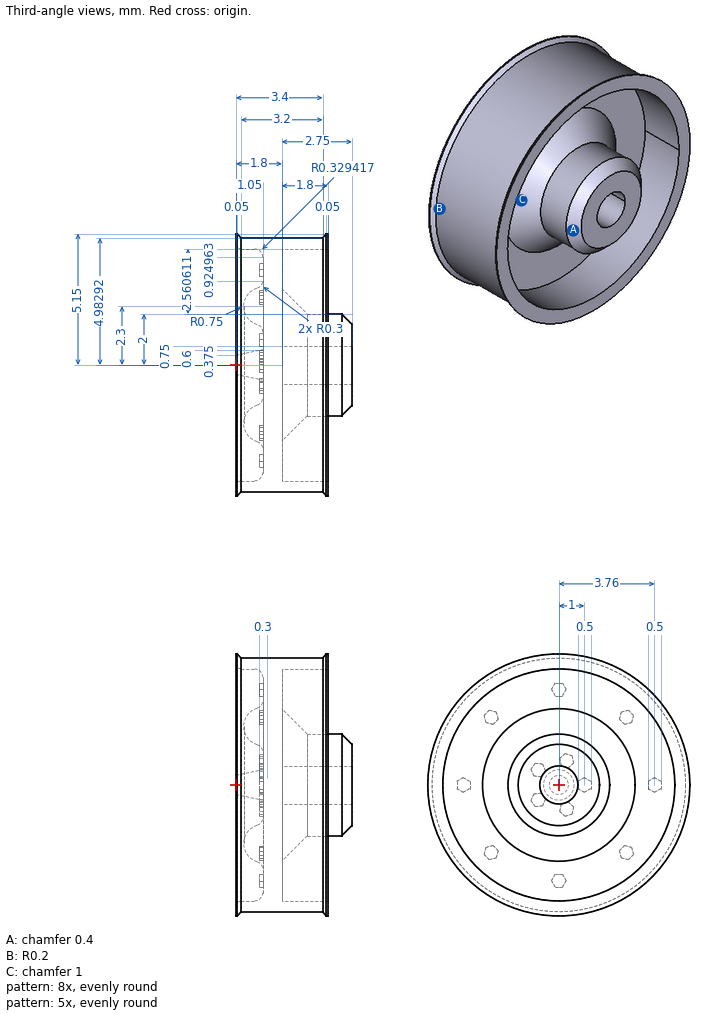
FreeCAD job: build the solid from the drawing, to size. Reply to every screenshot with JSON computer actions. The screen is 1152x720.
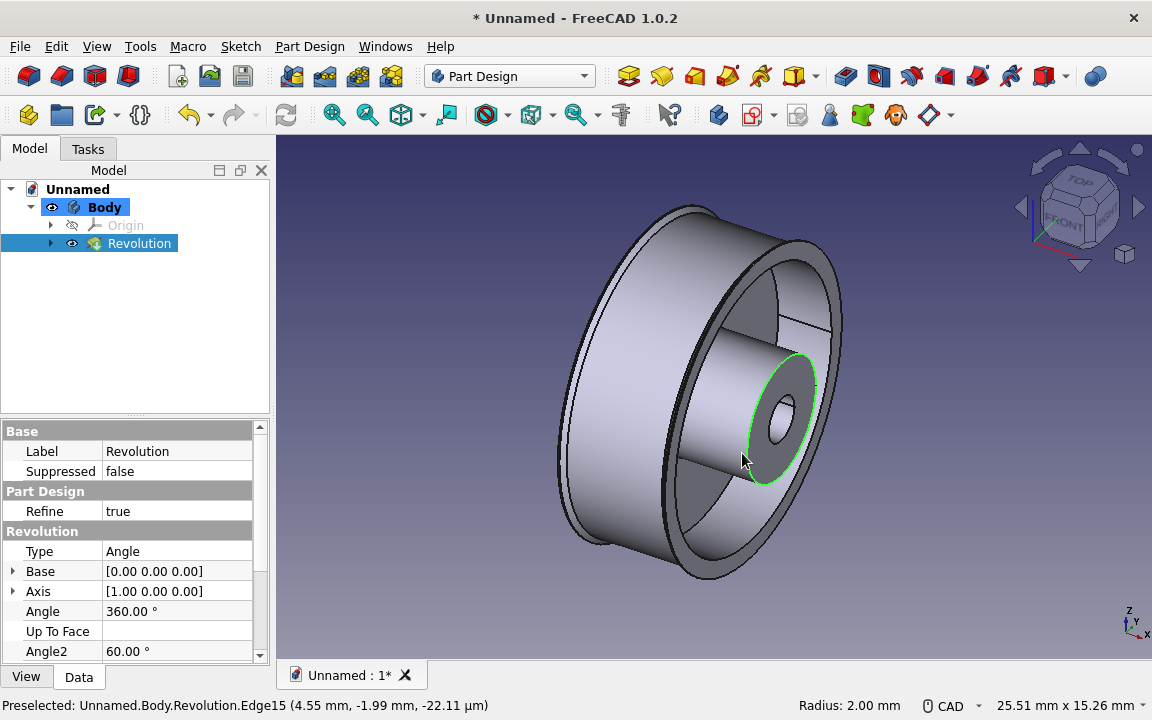
{"action": "left_click", "coordinate": [62, 76]}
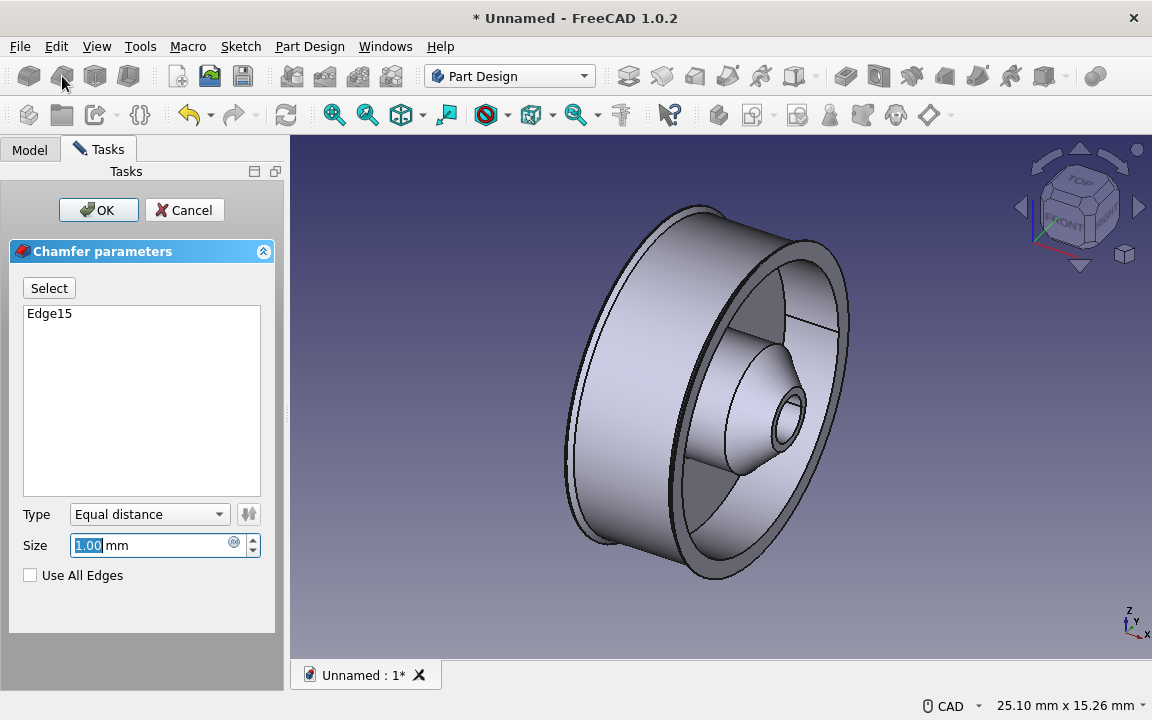
{"action": "type", "text": "0.4"}
{"action": "key", "text": "Tab"}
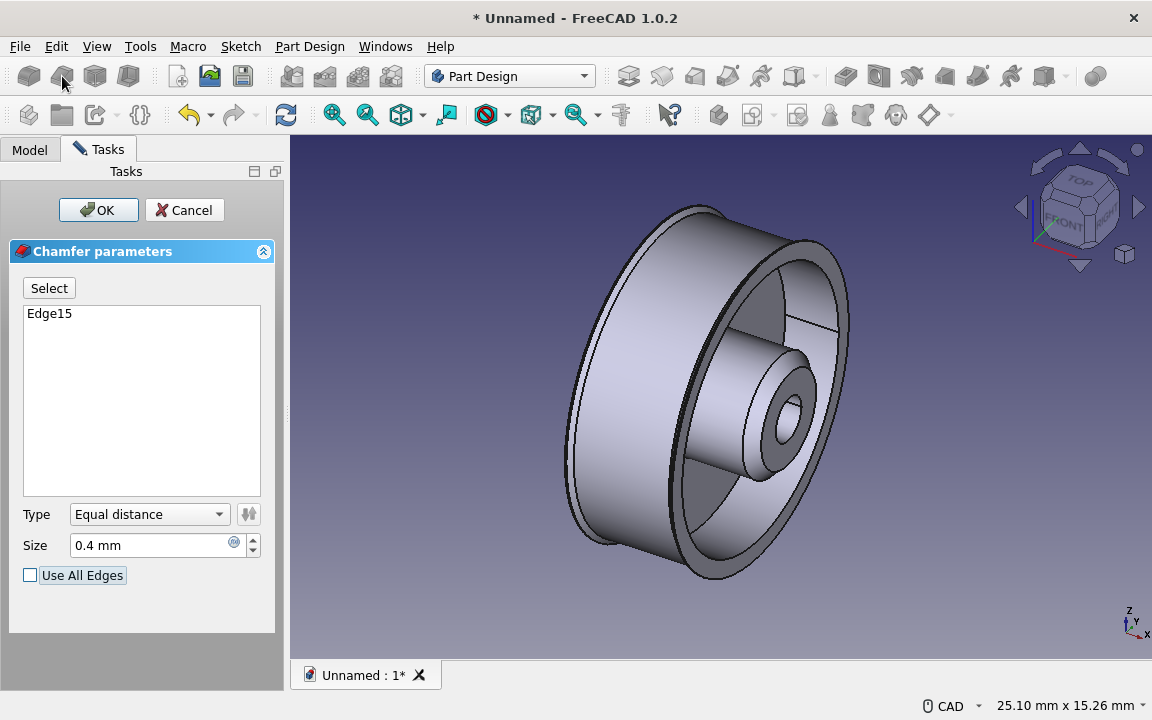
{"action": "left_click", "coordinate": [99, 210]}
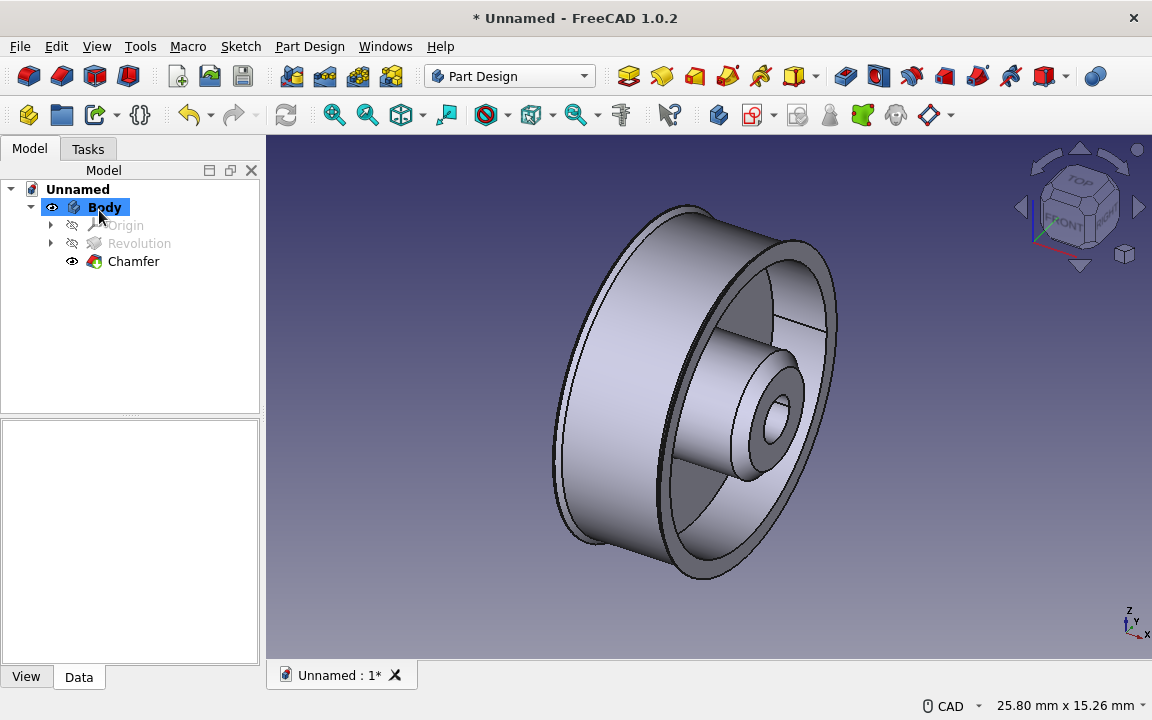
{"action": "key", "text": "0"}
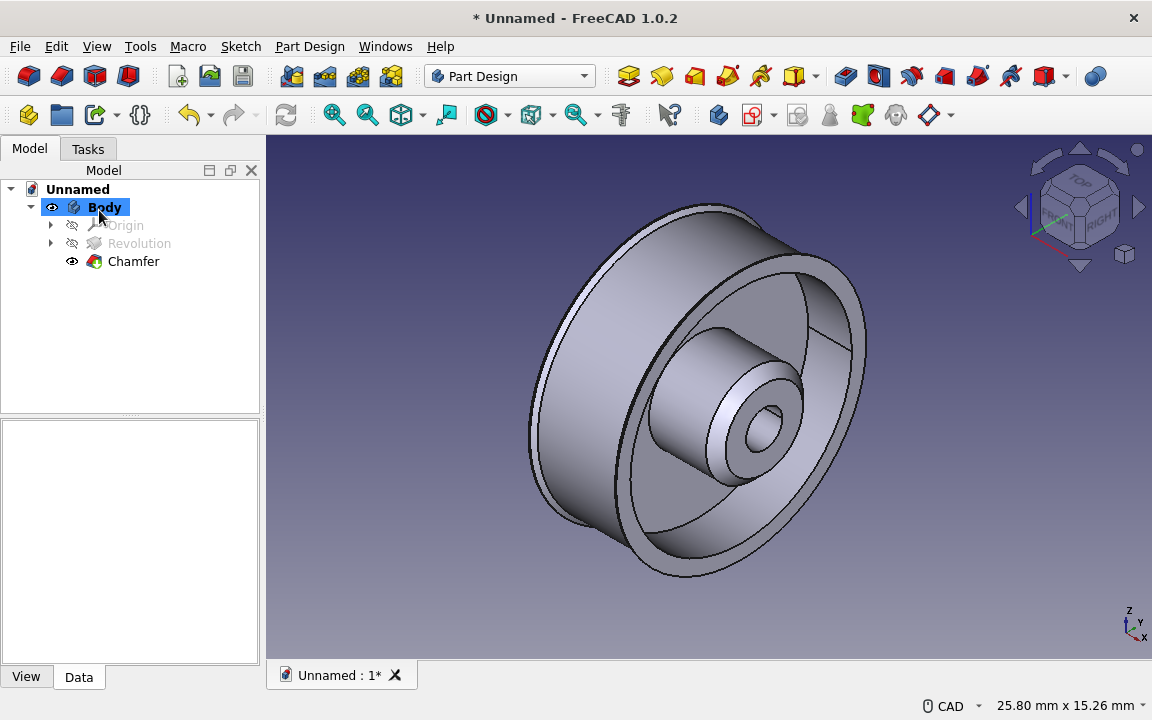
{"action": "key", "text": "2"}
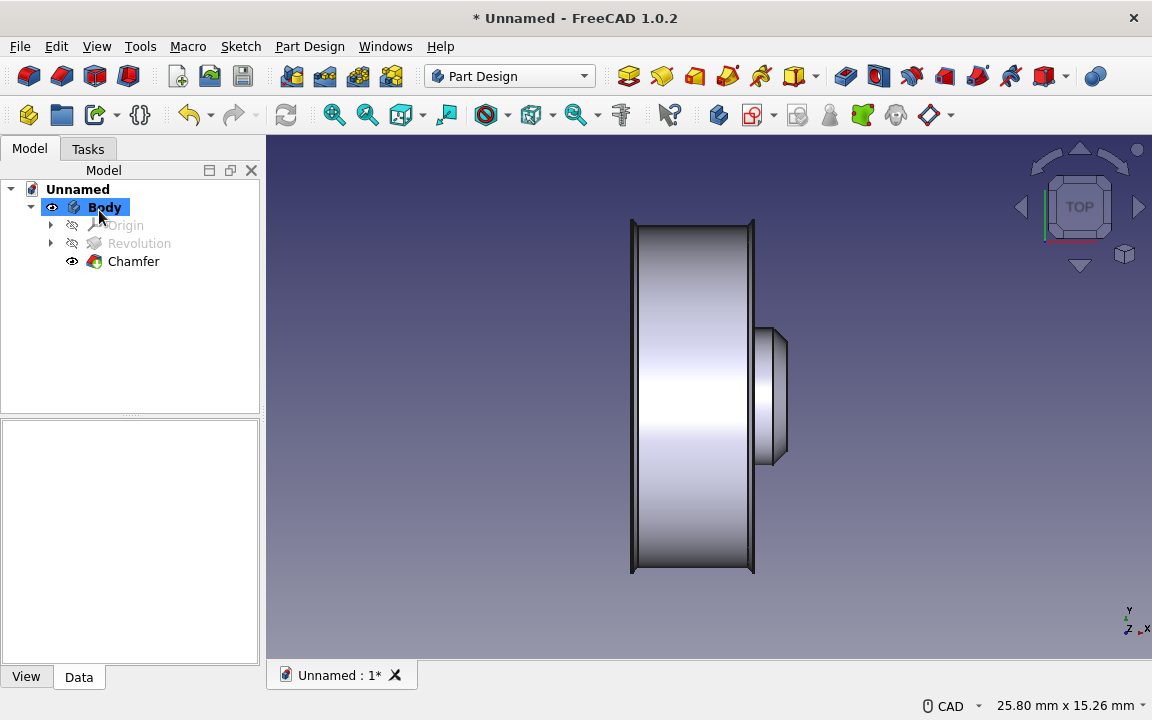
{"action": "key", "text": "1"}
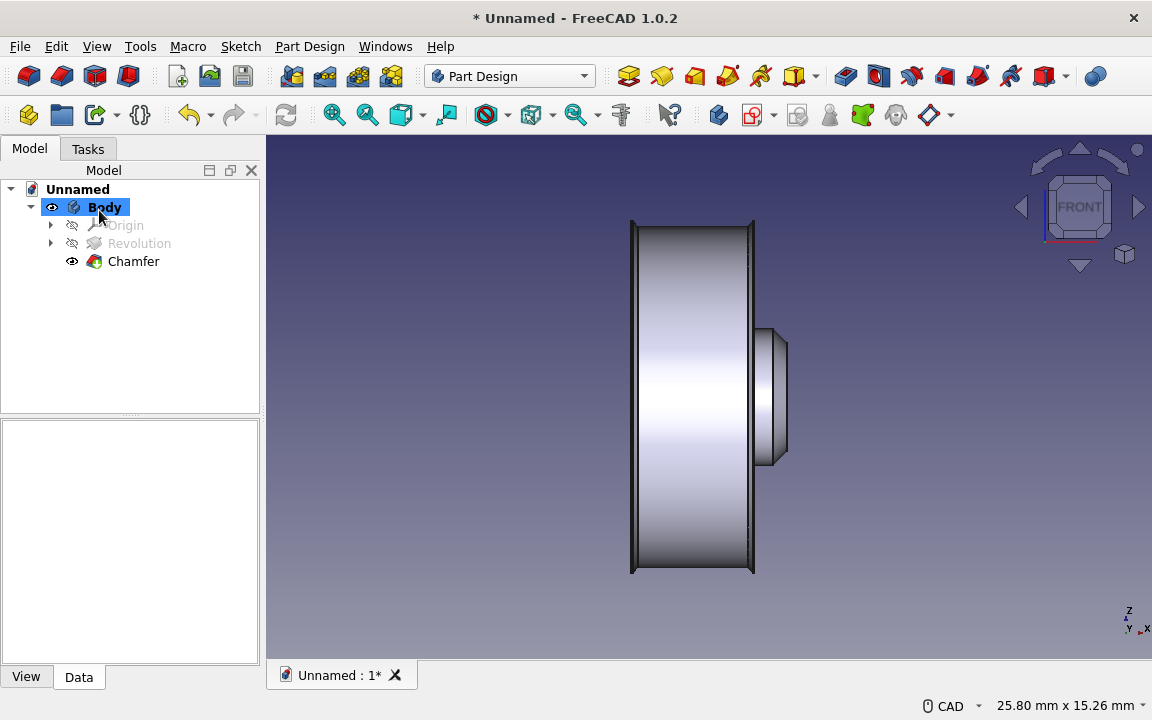
{"action": "key", "text": "3"}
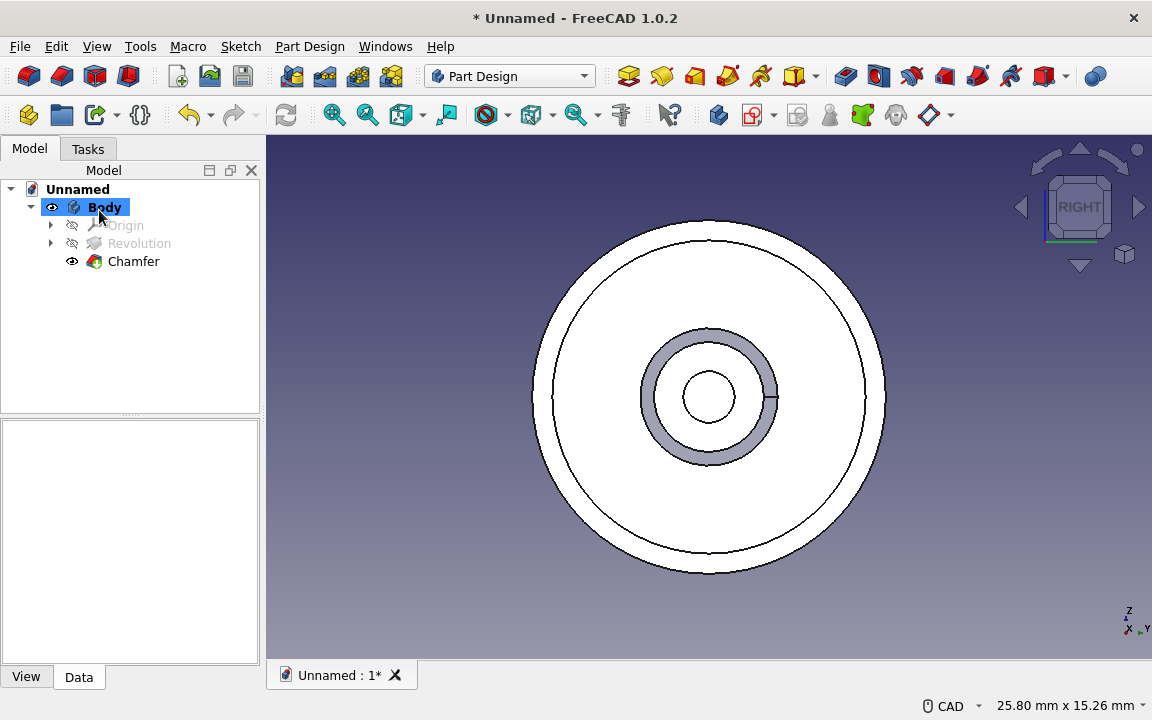
{"action": "key", "text": "5"}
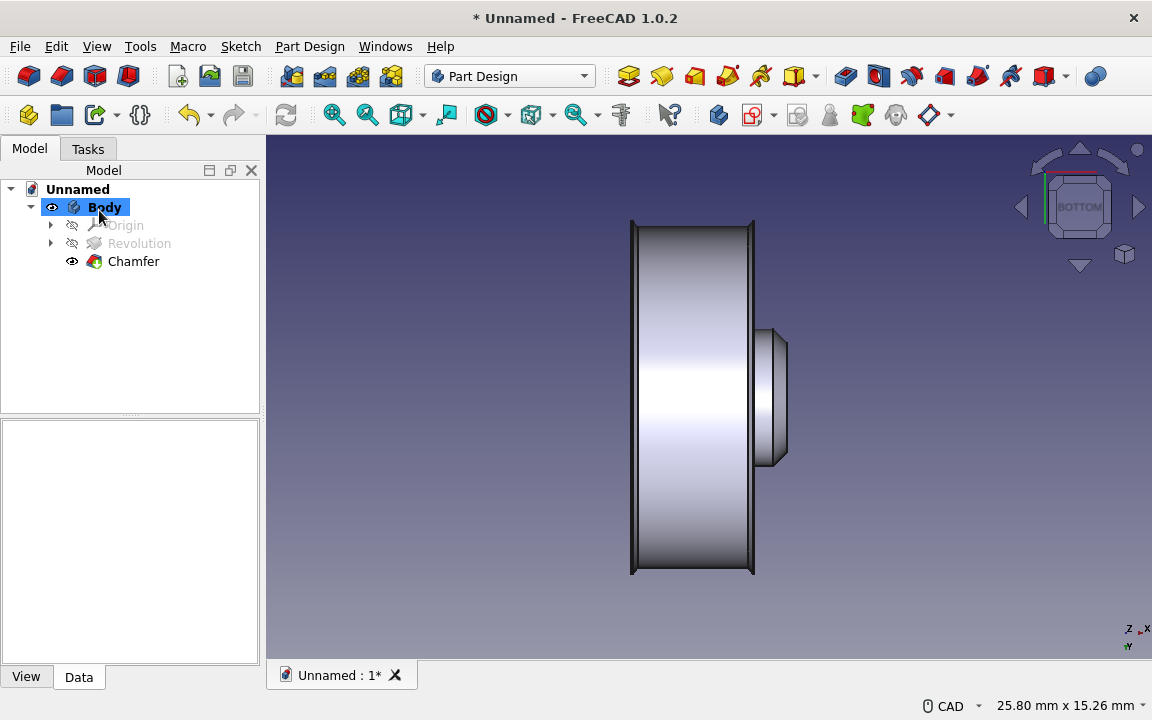
{"action": "key", "text": "4"}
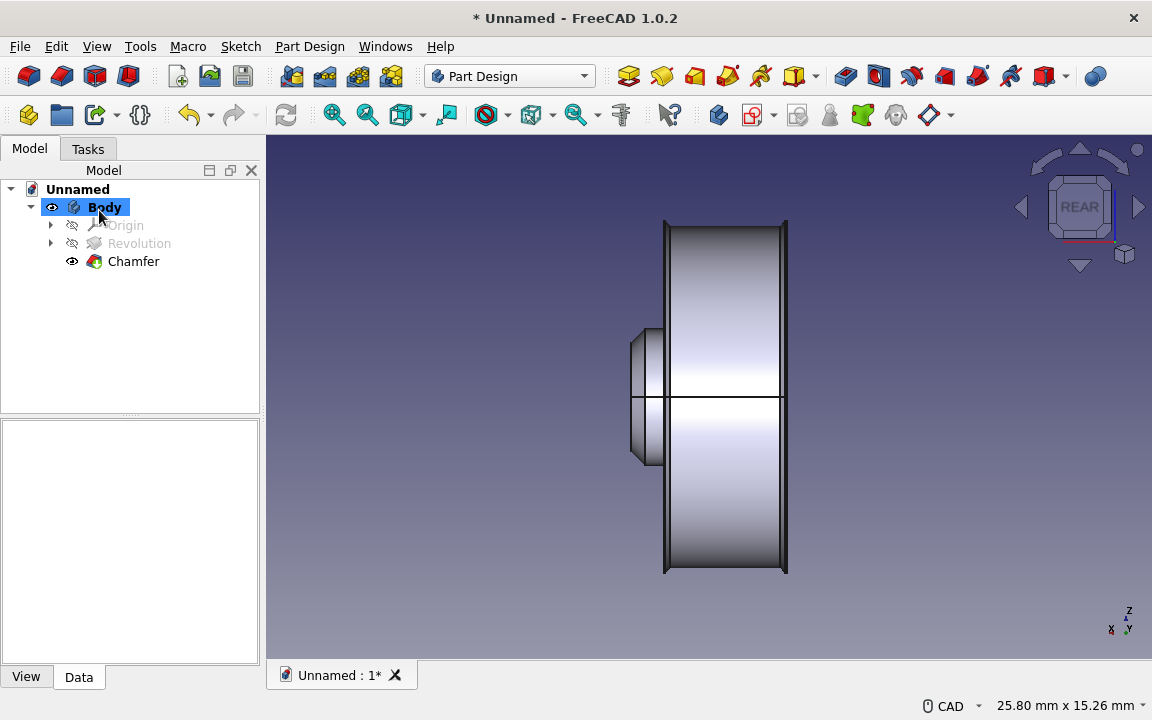
{"action": "key", "text": "6"}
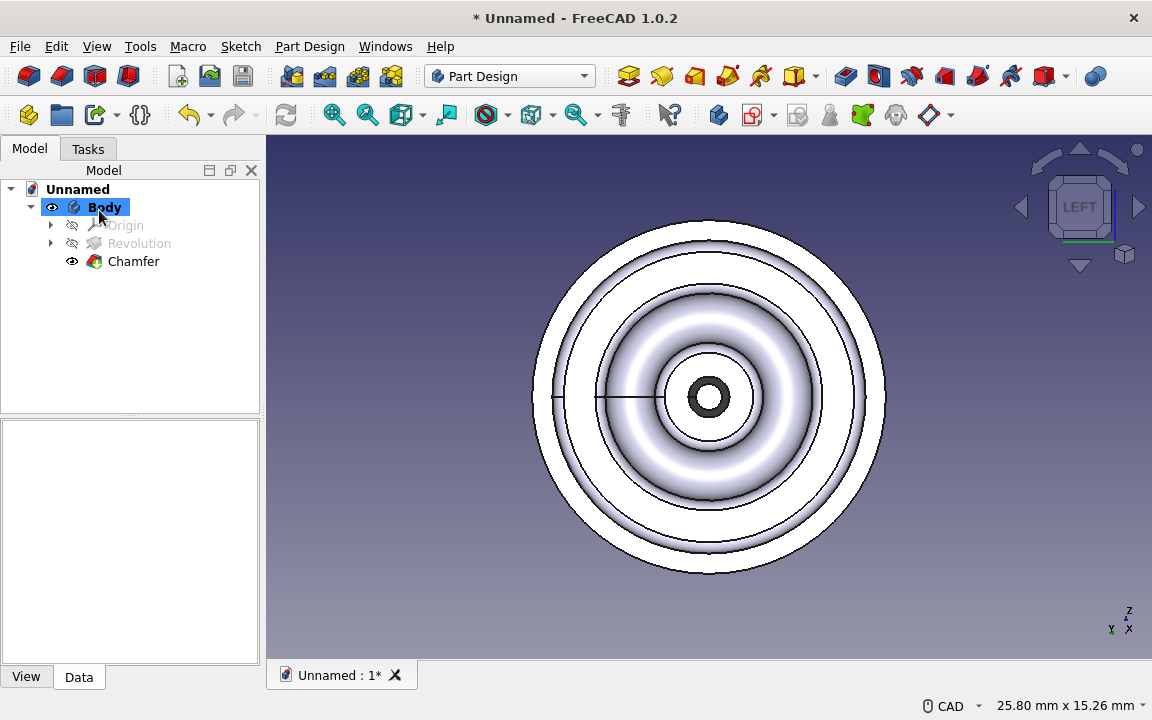
{"action": "left_click", "coordinate": [866, 396]}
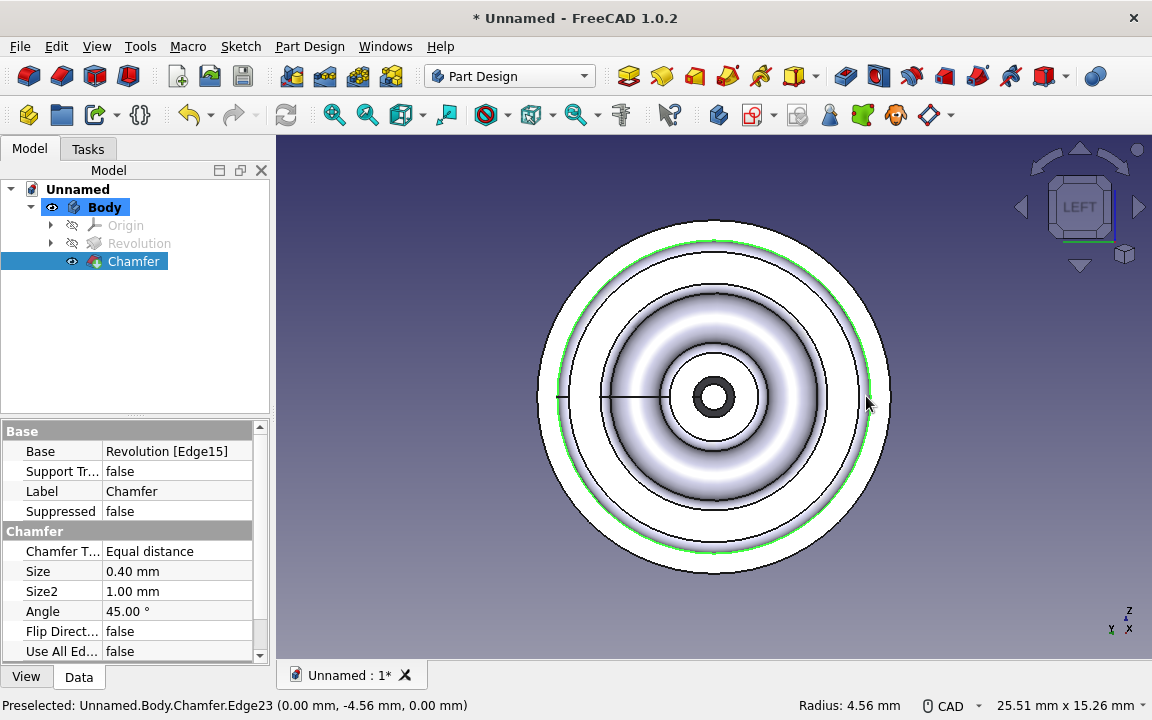
{"action": "left_click", "coordinate": [29, 76]}